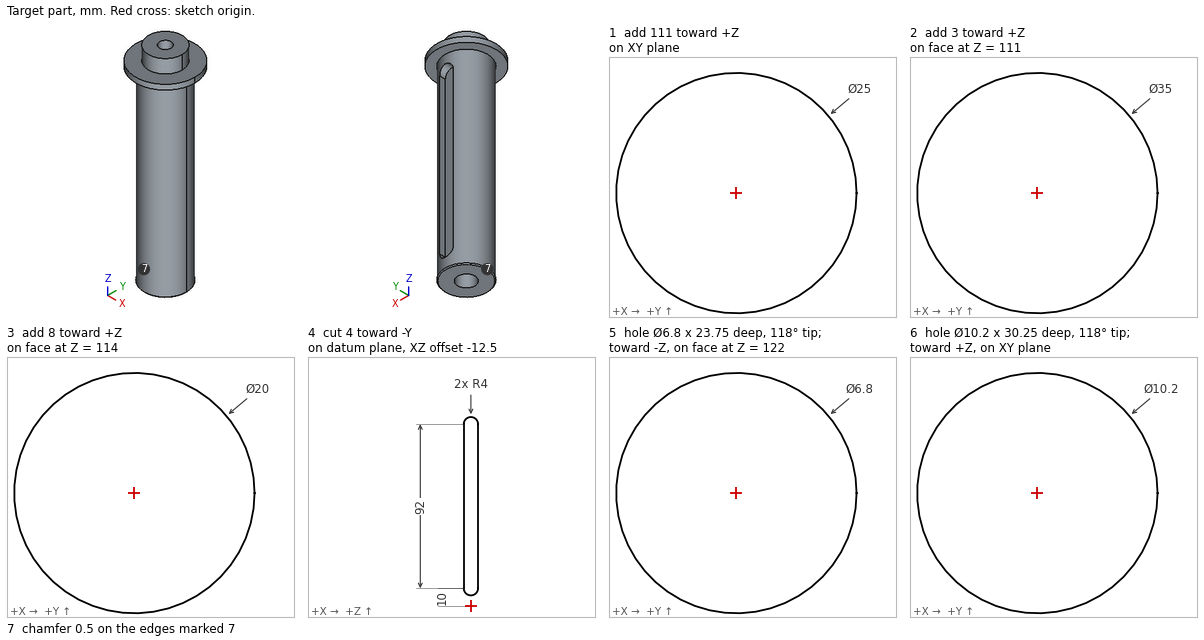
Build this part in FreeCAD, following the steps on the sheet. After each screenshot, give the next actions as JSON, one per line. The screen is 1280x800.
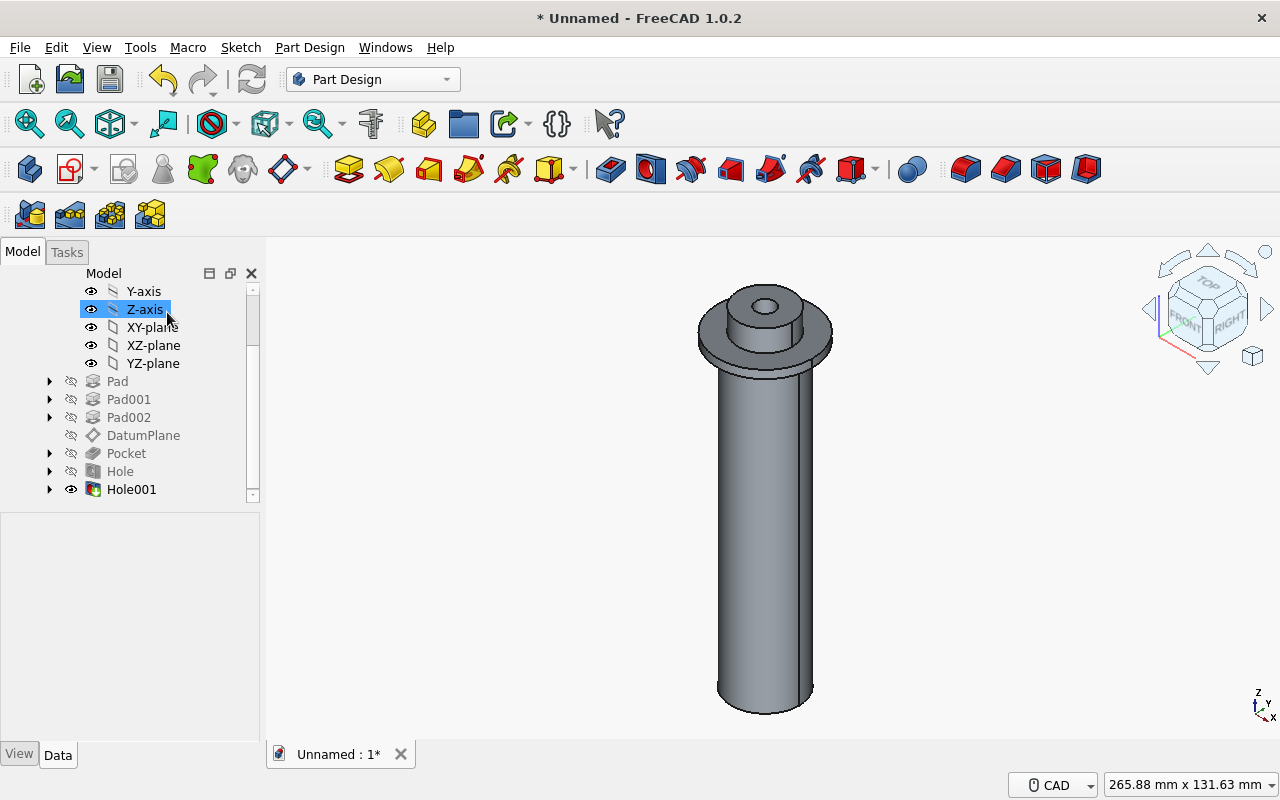
{"action": "left_click", "coordinate": [30, 124]}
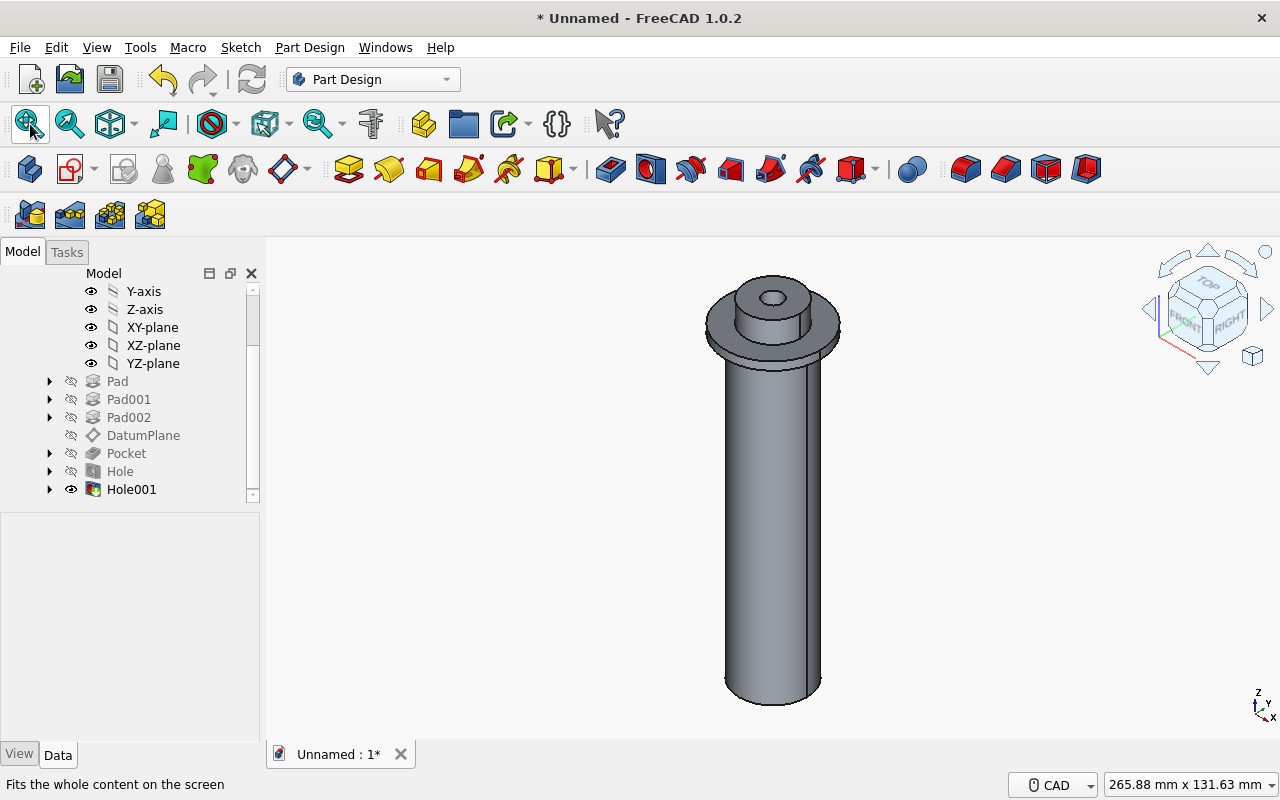
{"action": "key", "text": "2"}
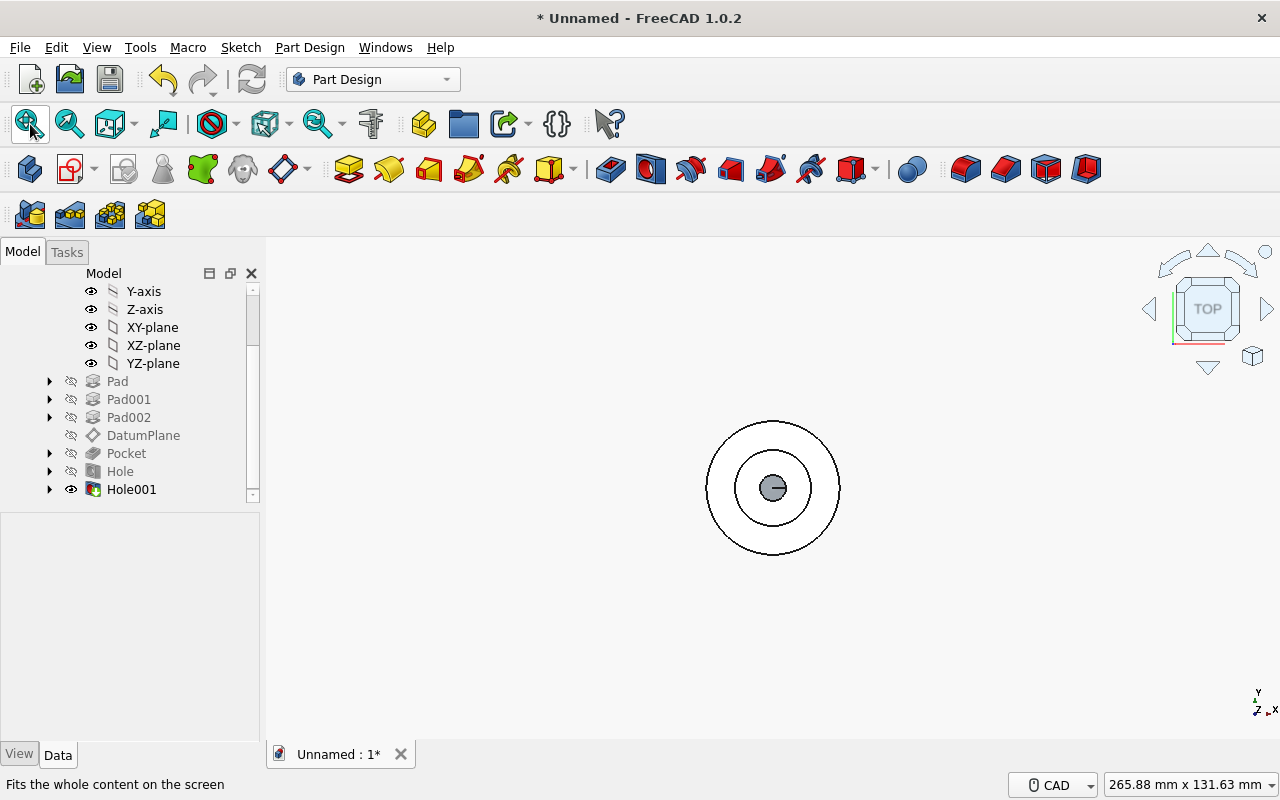
{"action": "key", "text": "v f"}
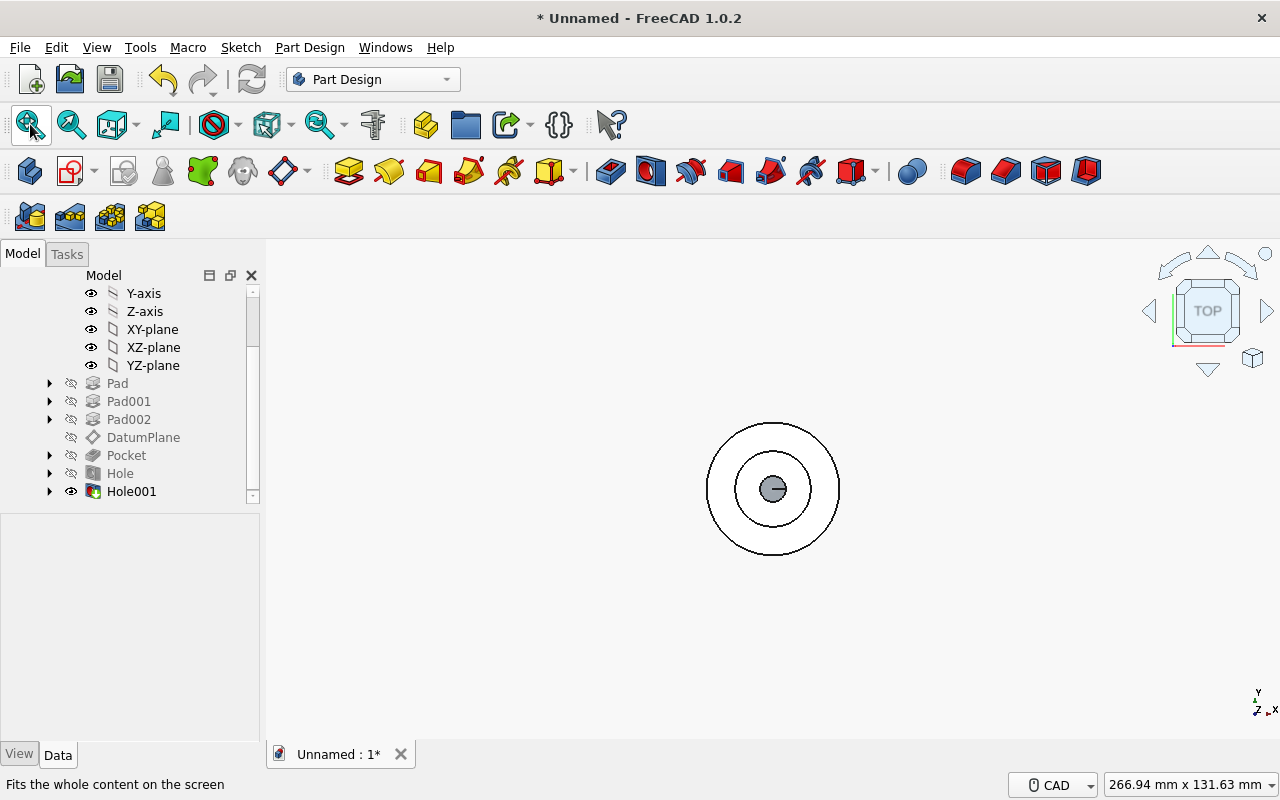
{"action": "key", "text": "1"}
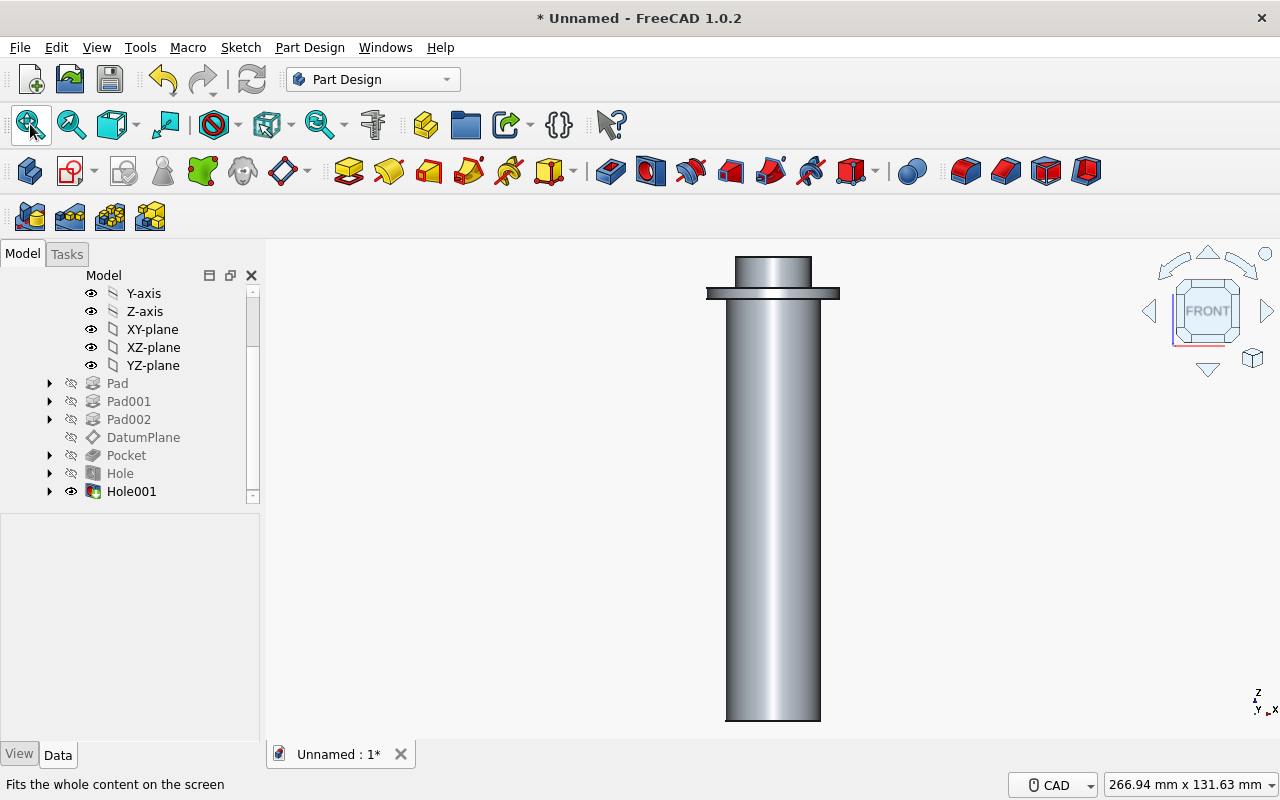
{"action": "key", "text": "3"}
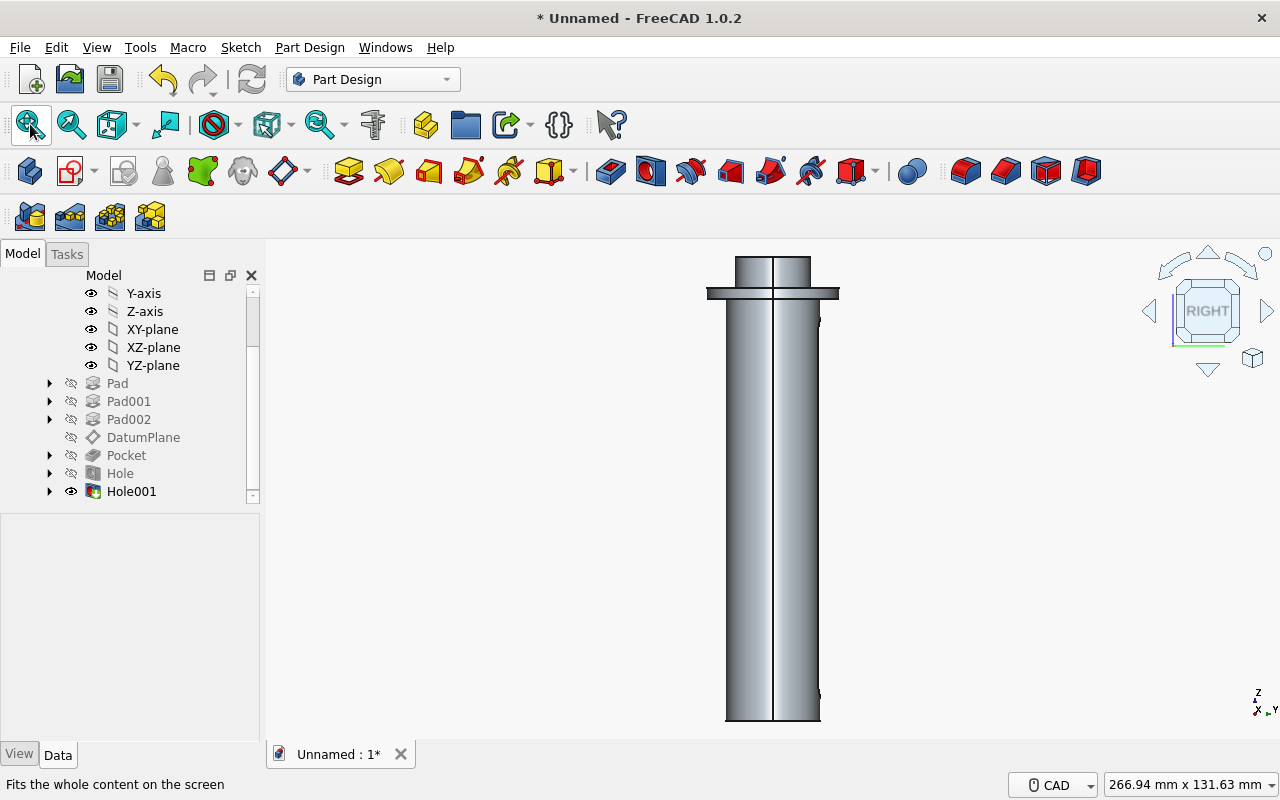
{"action": "key", "text": "5"}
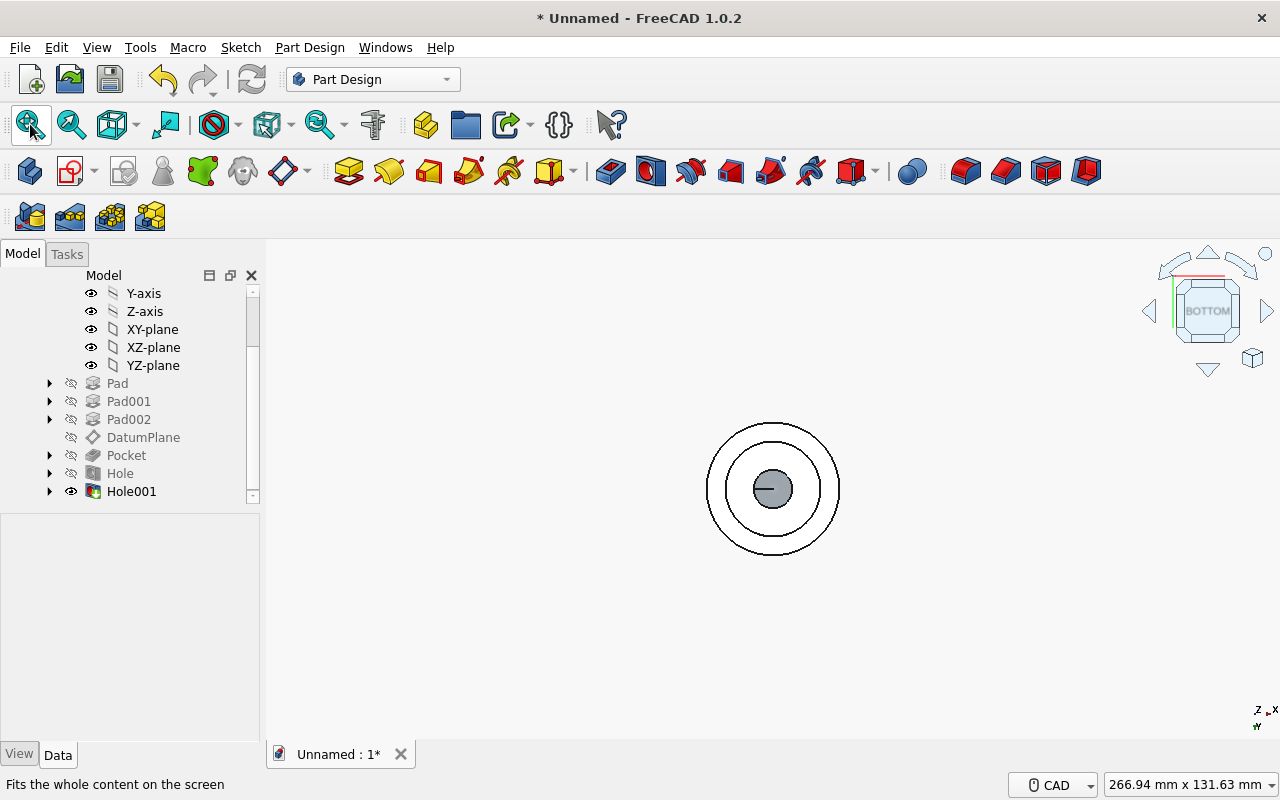
{"action": "left_click", "coordinate": [32, 126]}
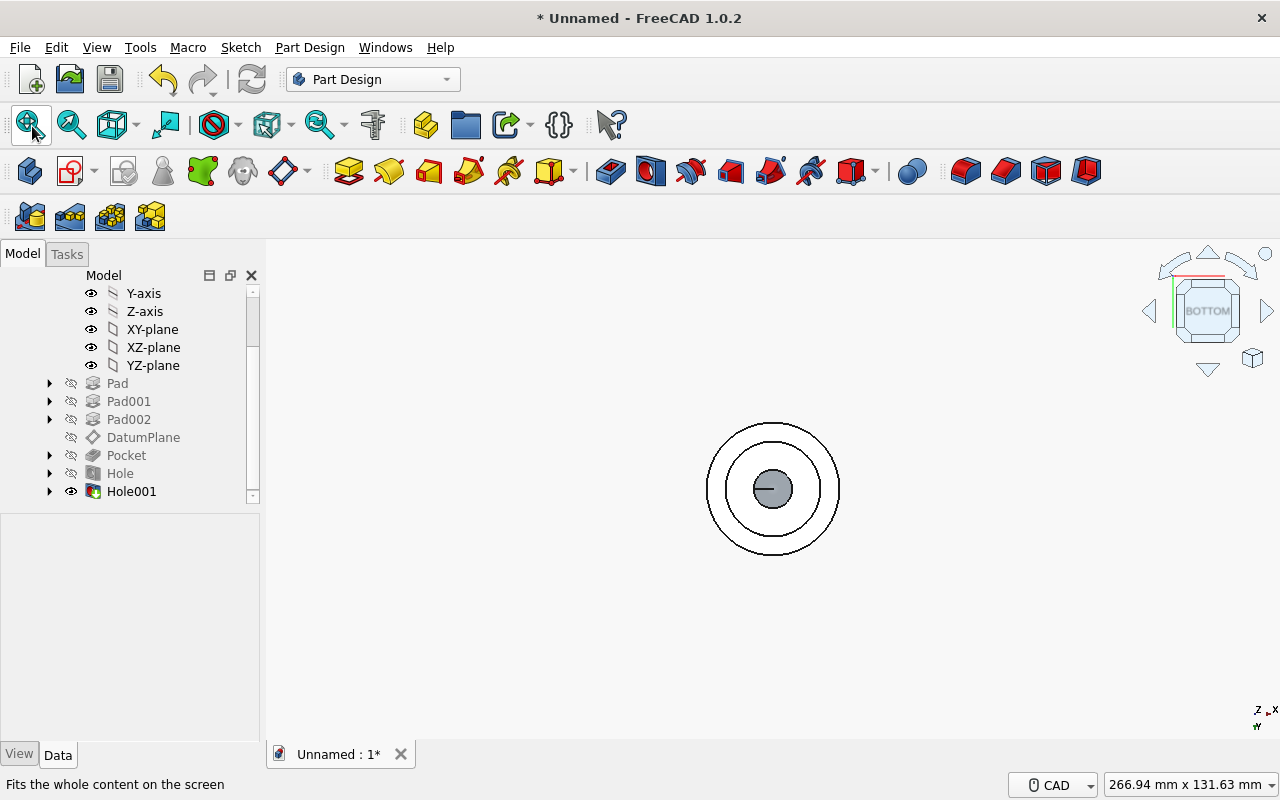
{"action": "left_click", "coordinate": [726, 488]}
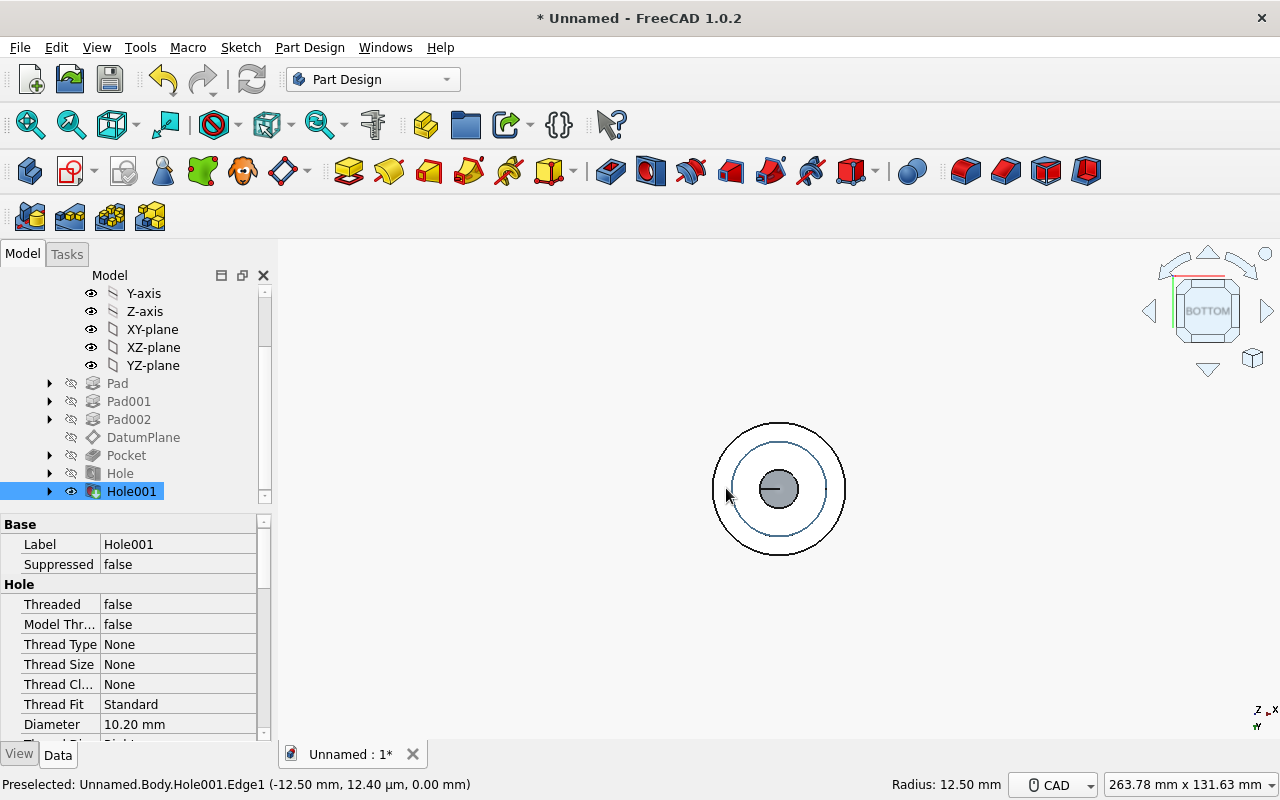
{"action": "left_click", "coordinate": [1006, 172]}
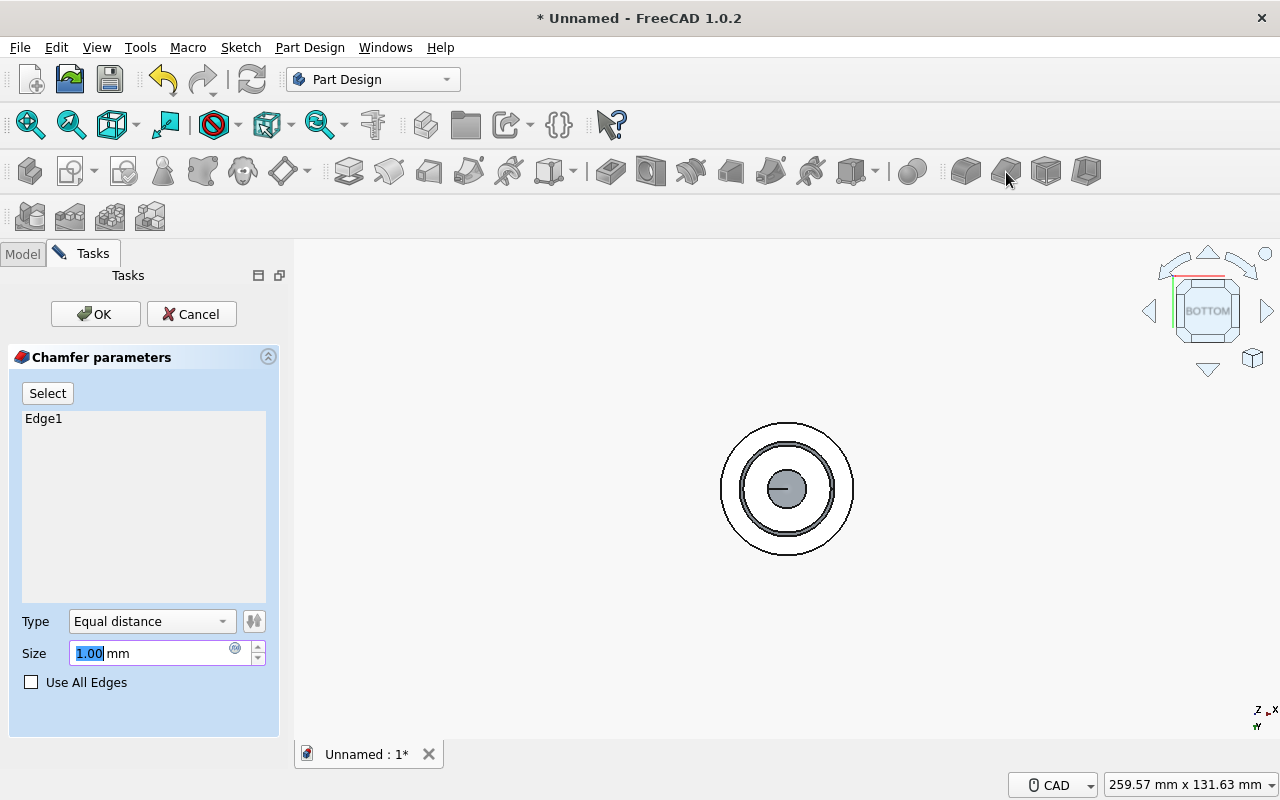
{"action": "type", "text": "0.5"}
{"action": "key", "text": "Tab"}